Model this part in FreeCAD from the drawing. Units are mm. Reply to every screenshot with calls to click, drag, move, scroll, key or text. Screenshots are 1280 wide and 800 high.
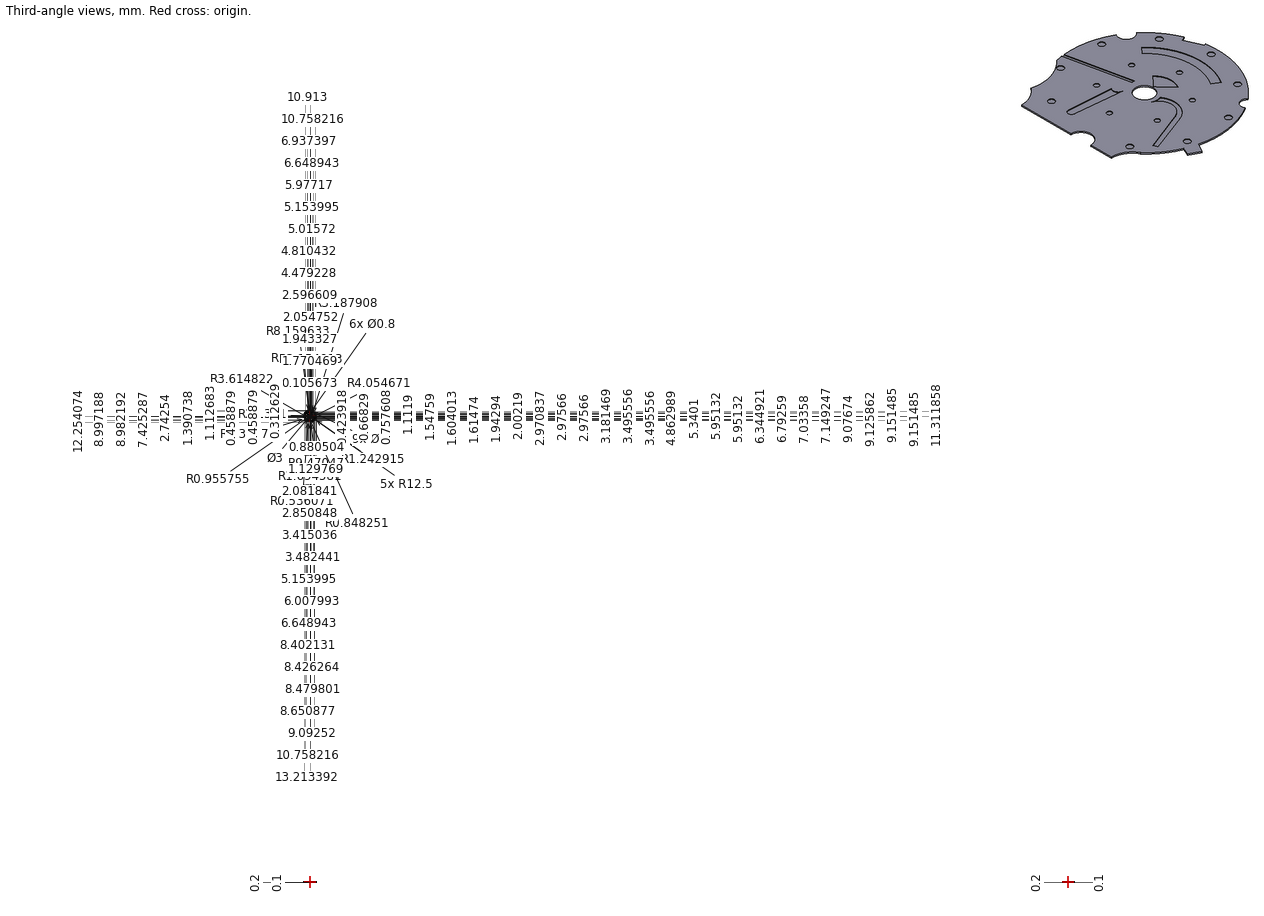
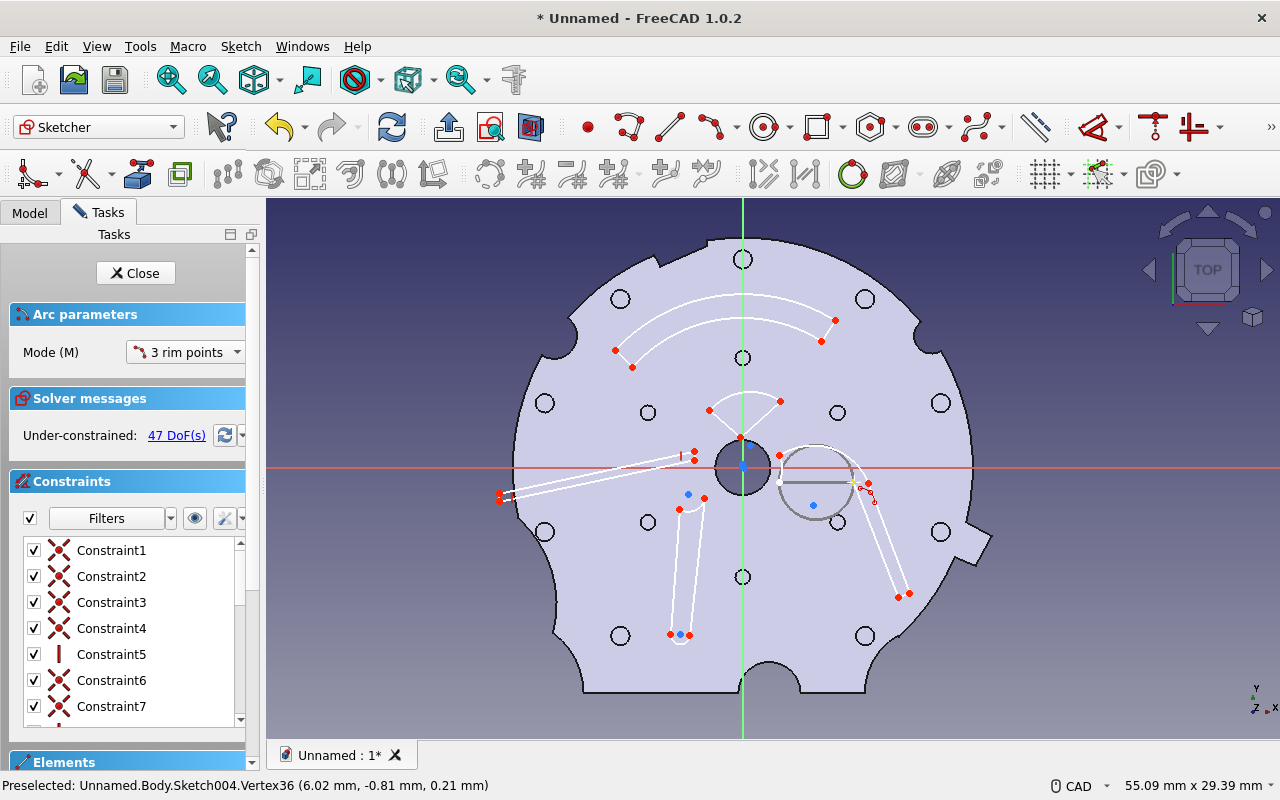
scroll(816, 456, up, 2)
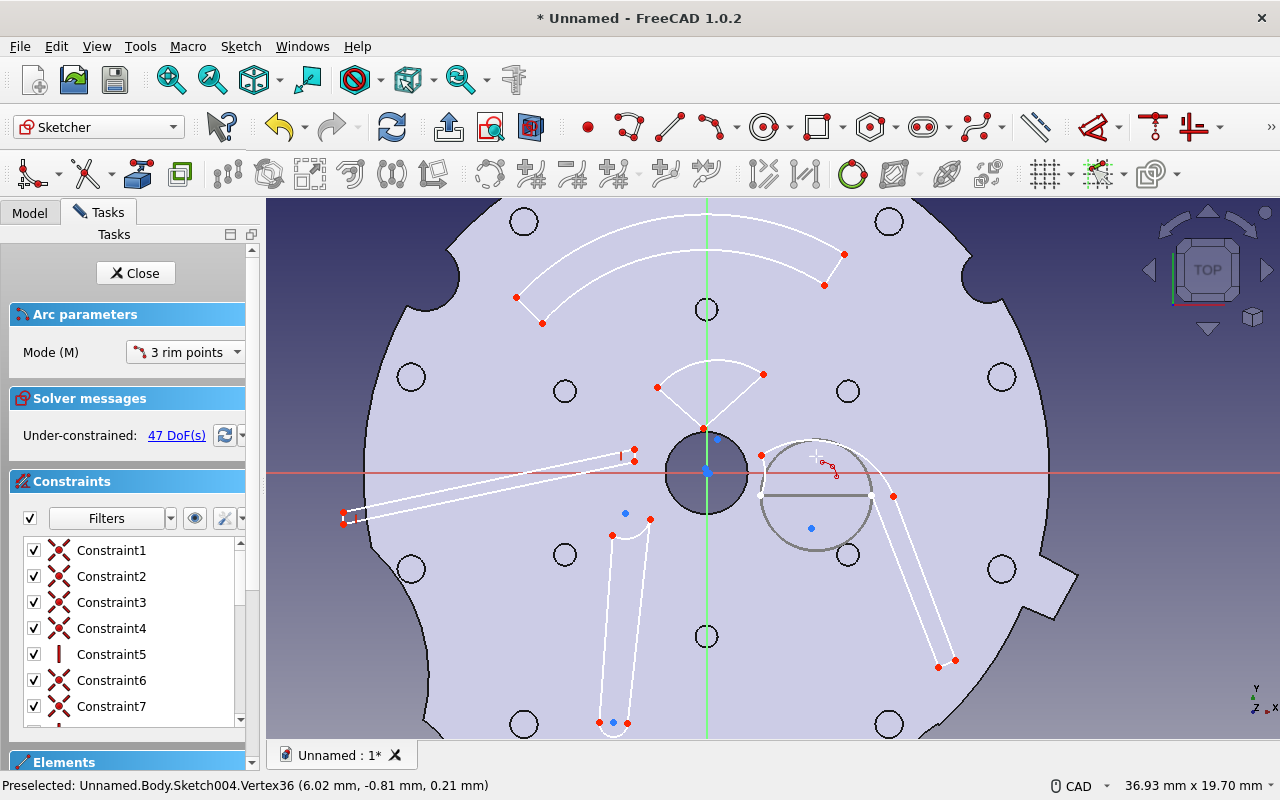
click(816, 456)
key(Escape)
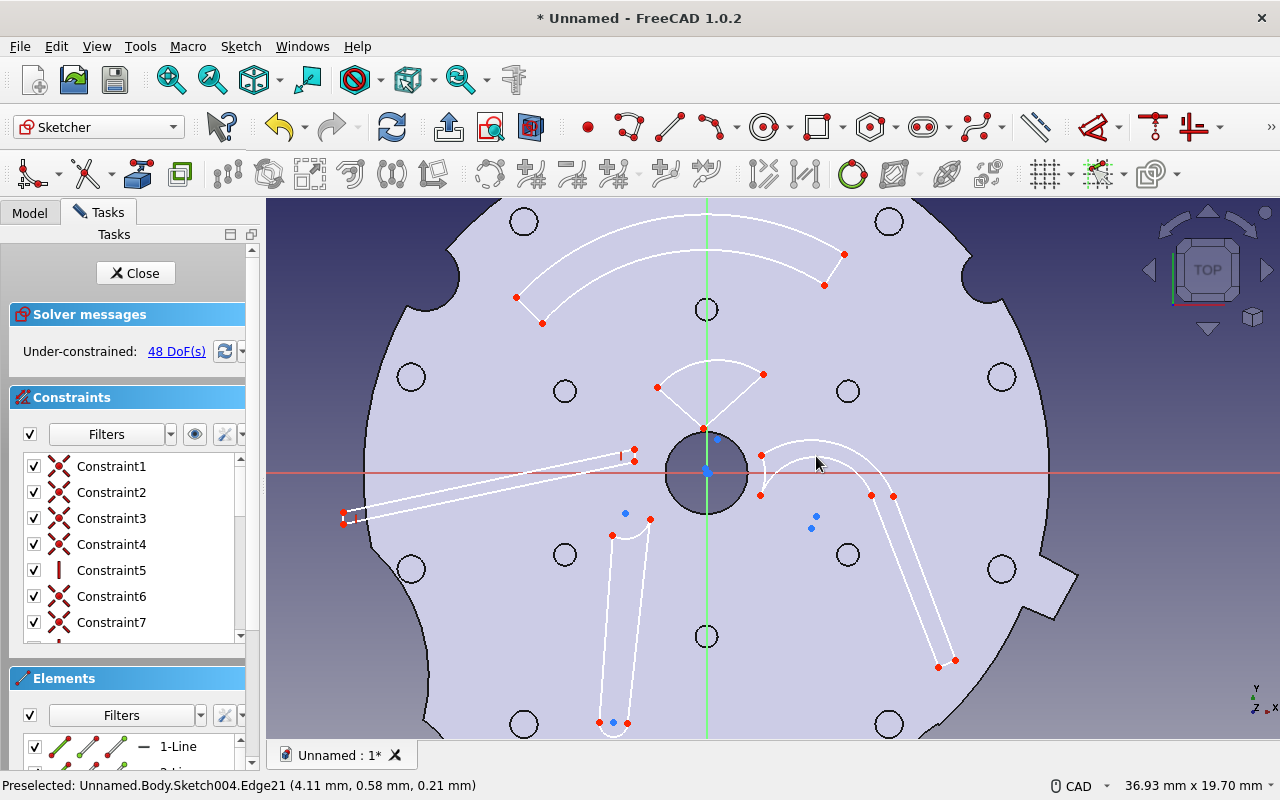
click(634, 662)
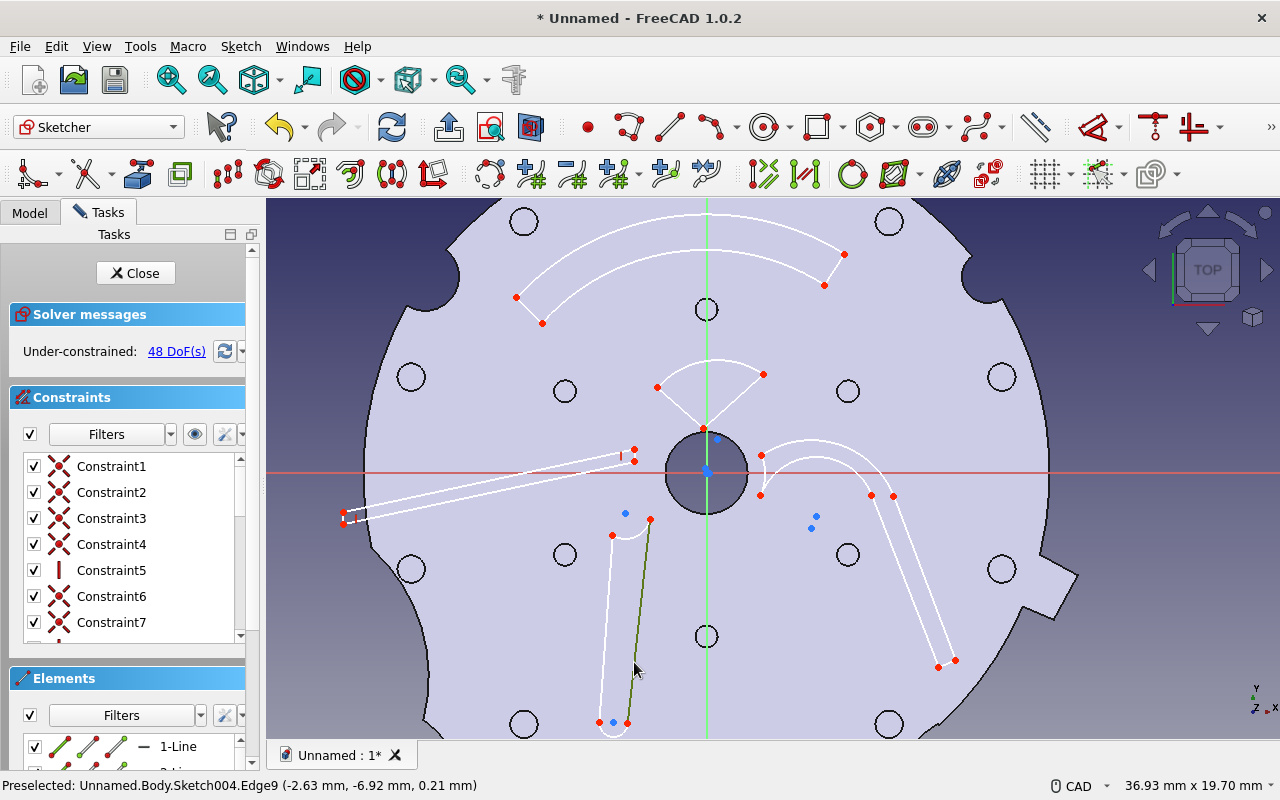
click(626, 539)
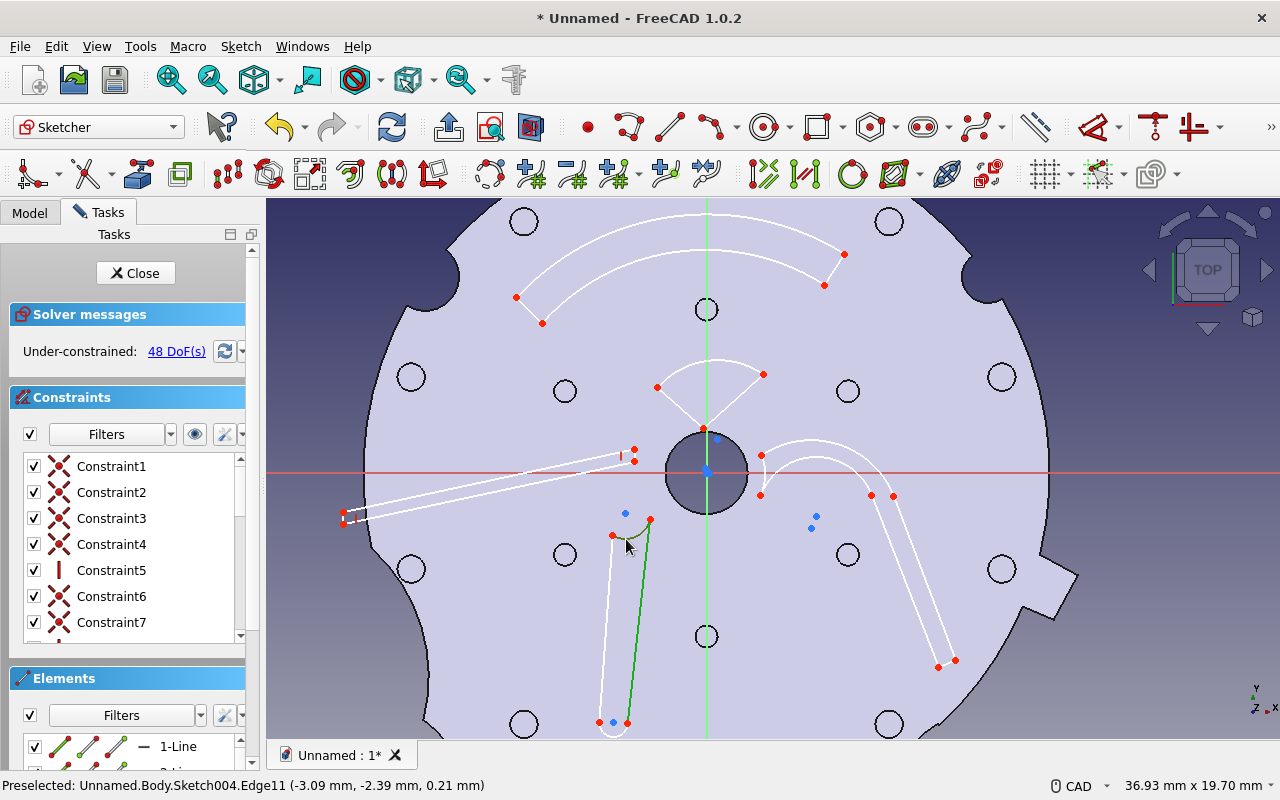
key(t)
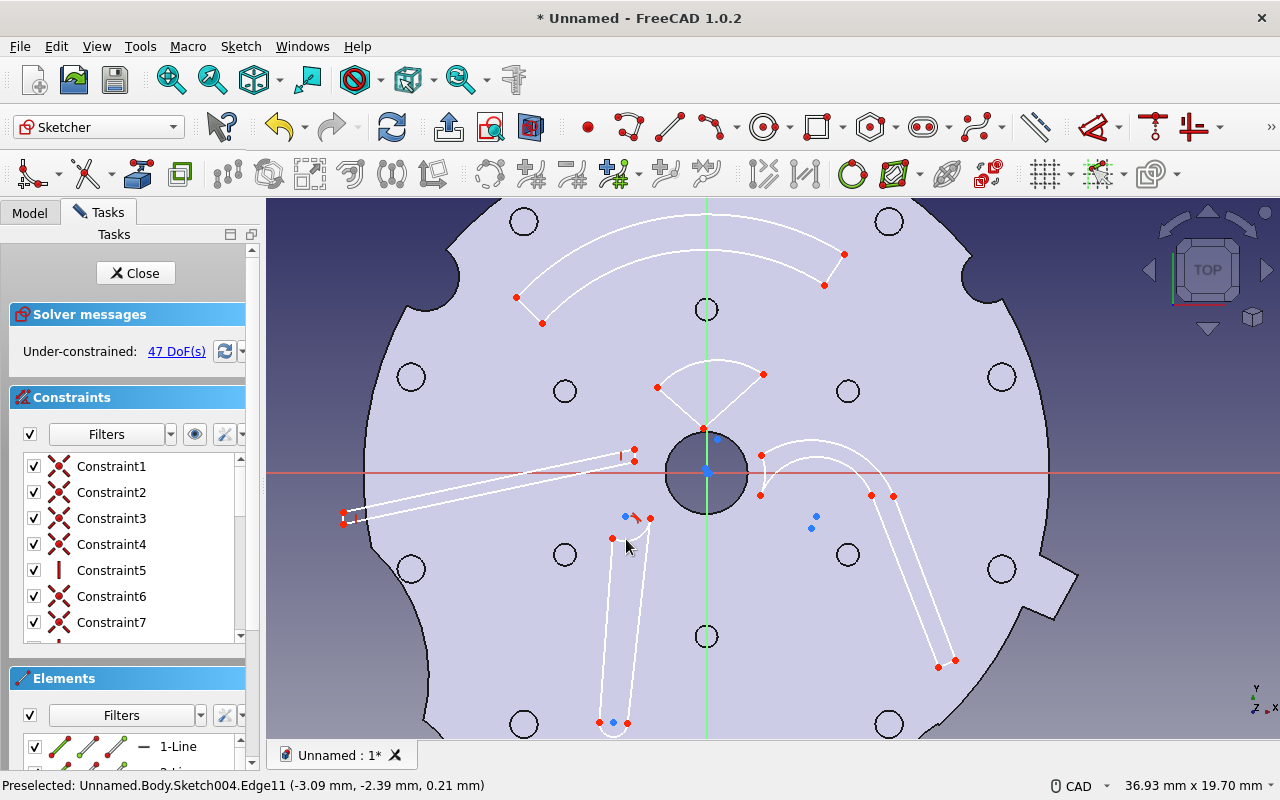
click(609, 593)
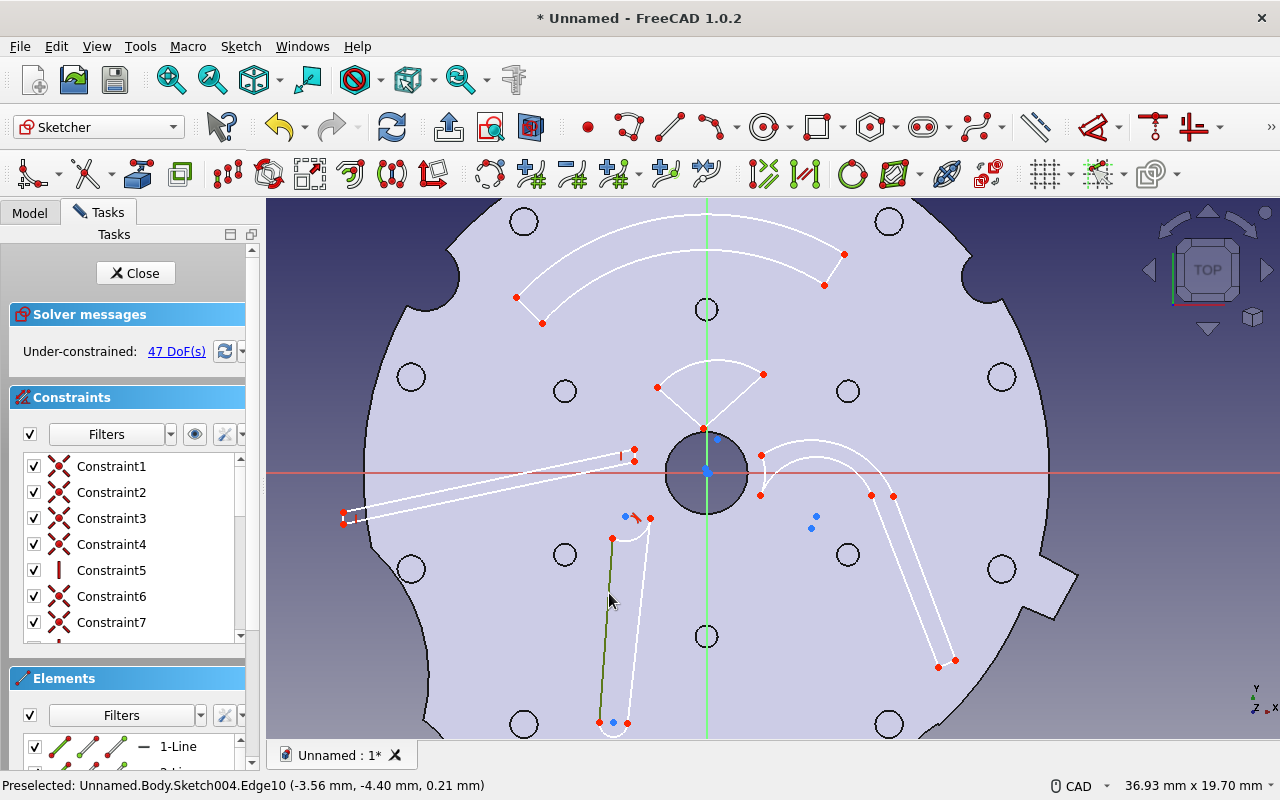
scroll(815, 454, down, 2)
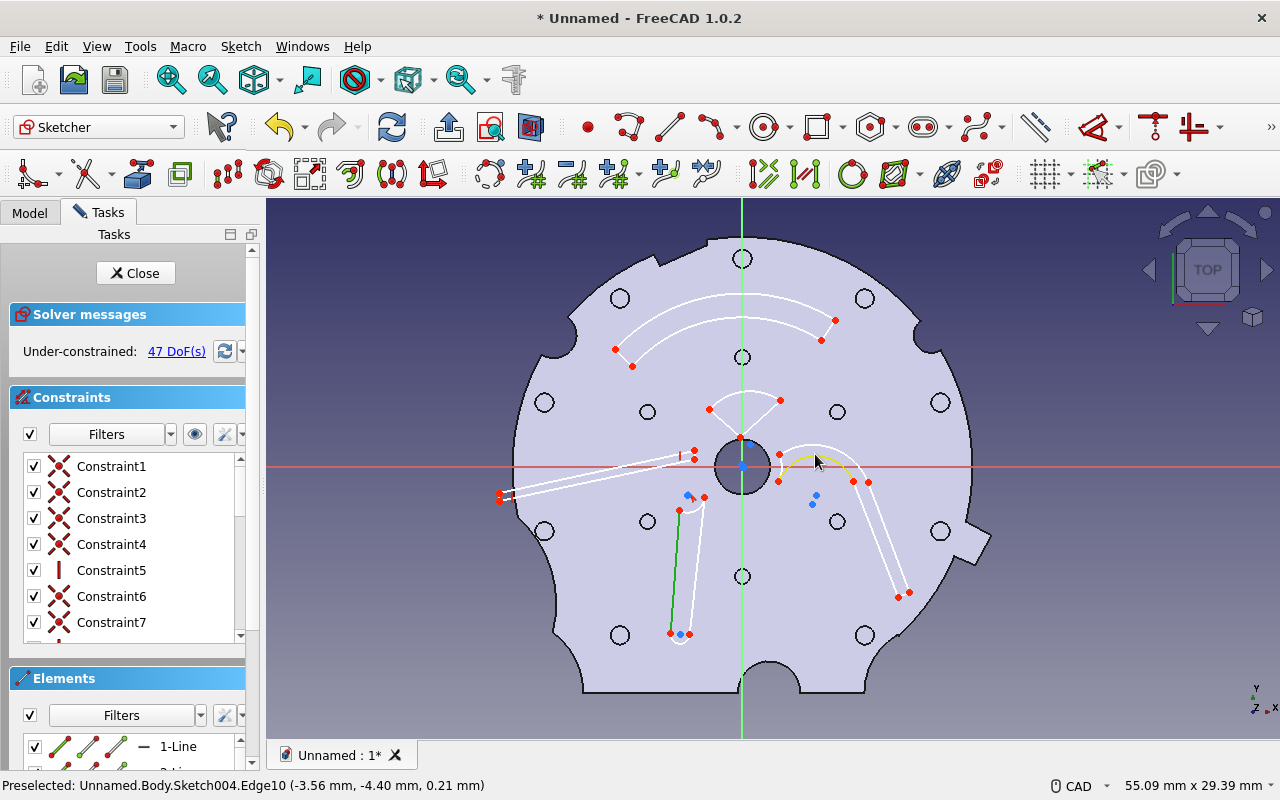
scroll(674, 642, up, 3)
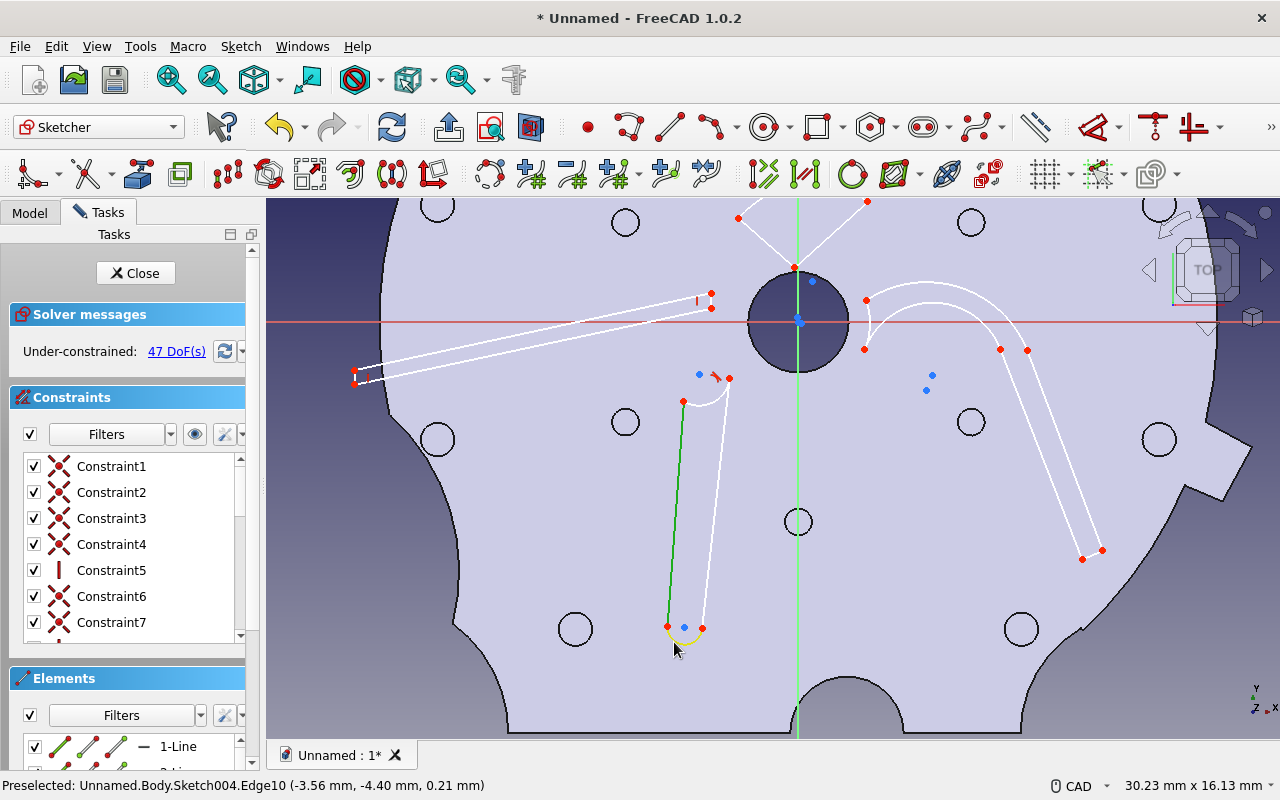
click(674, 641)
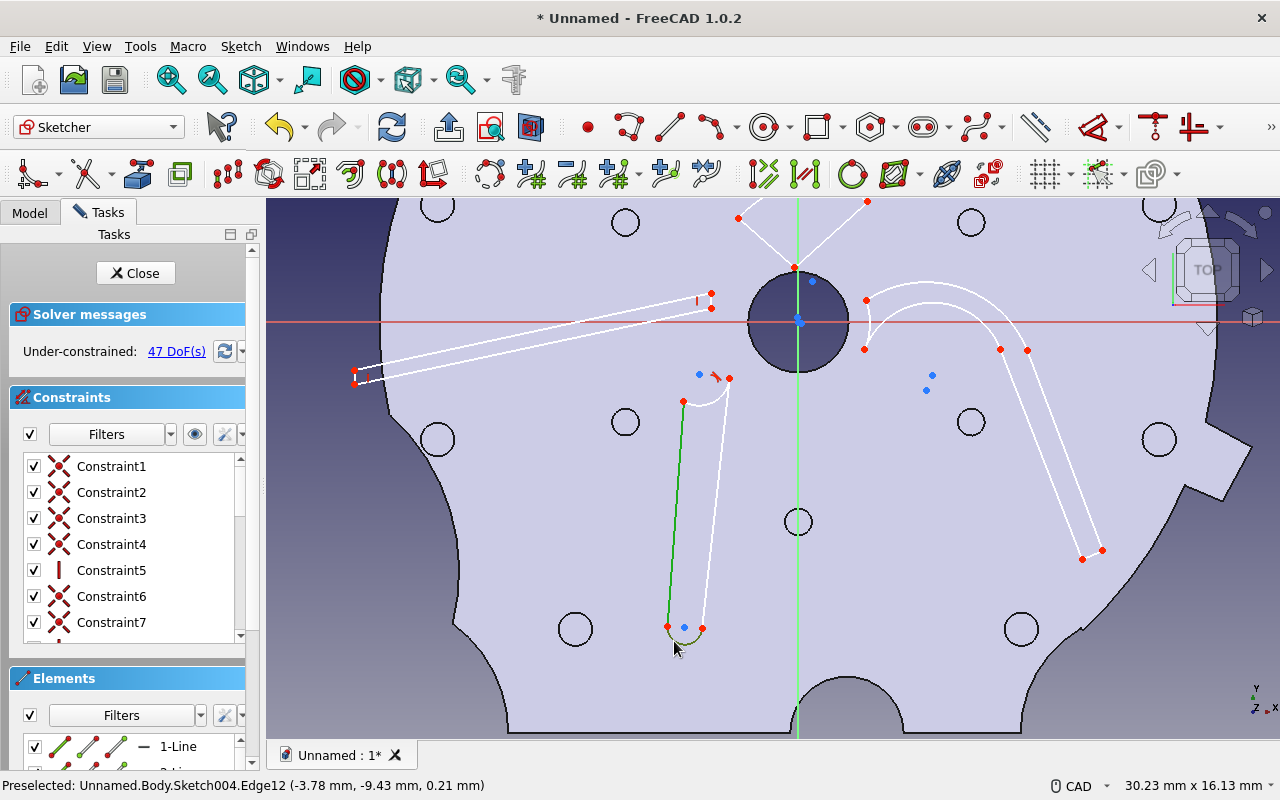
key(t)